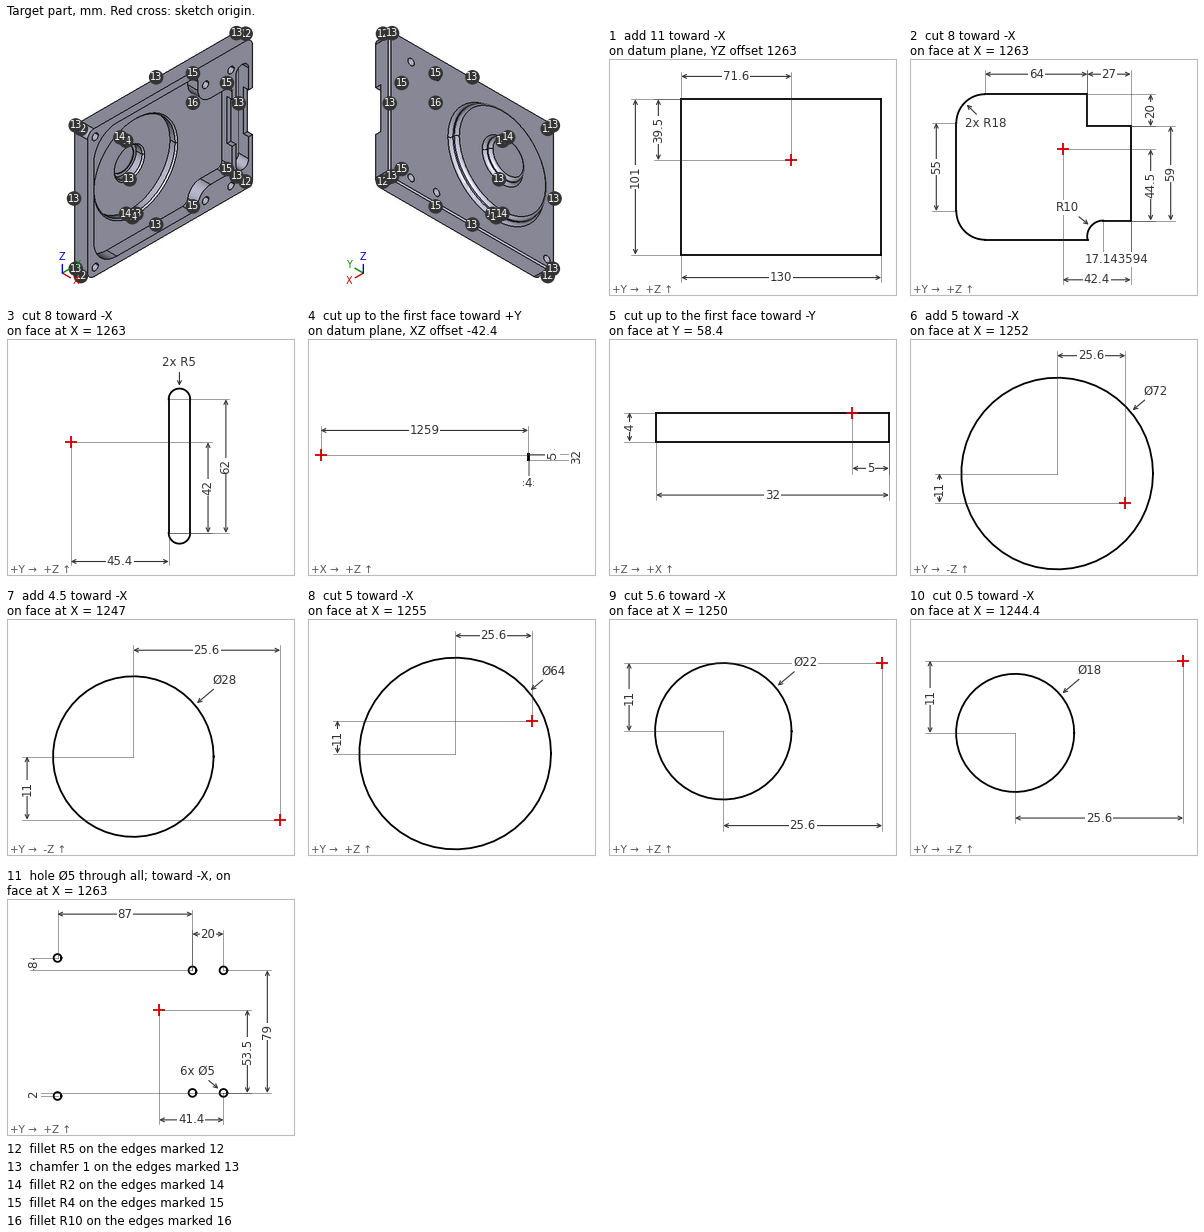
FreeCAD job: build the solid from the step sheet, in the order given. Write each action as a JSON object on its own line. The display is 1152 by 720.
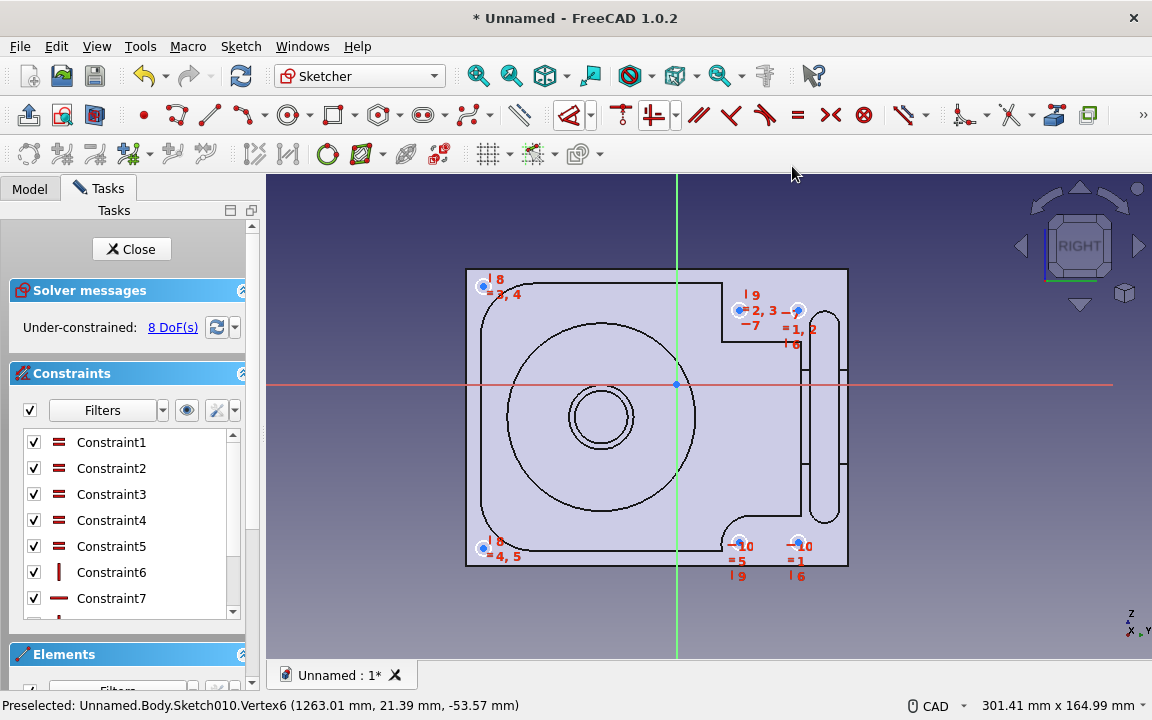
{"action": "scroll", "coordinate": [804, 548], "scroll_direction": "up", "scroll_amount": 5}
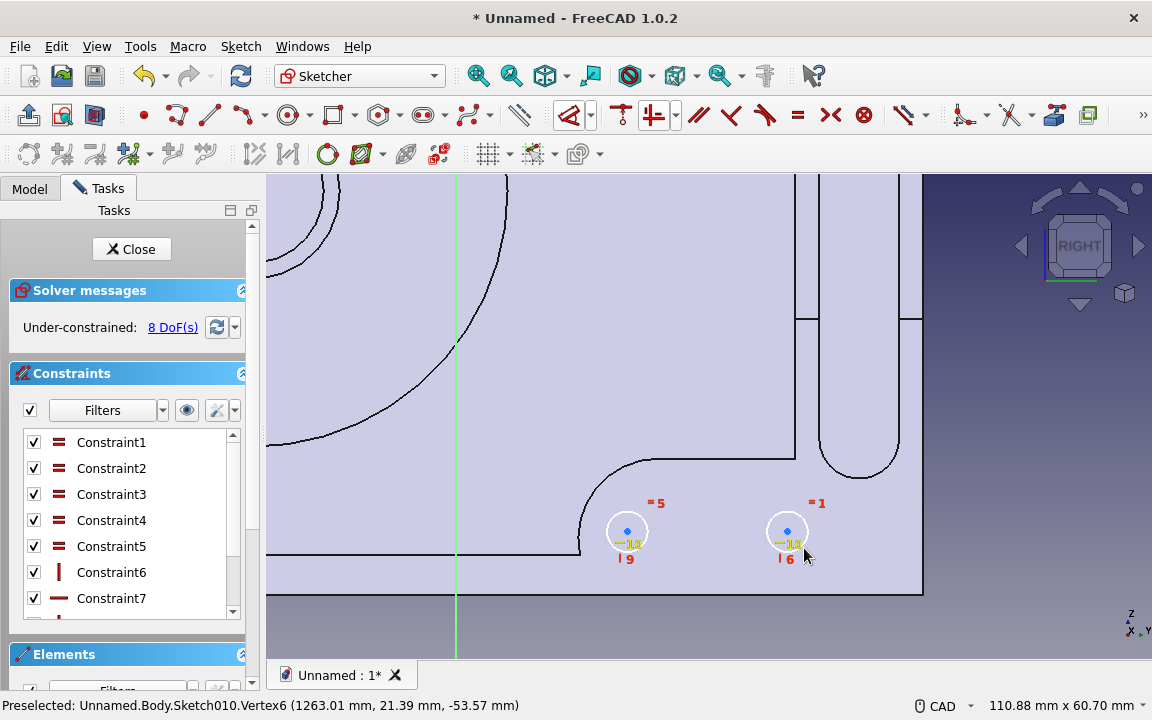
{"action": "left_click", "coordinate": [802, 546]}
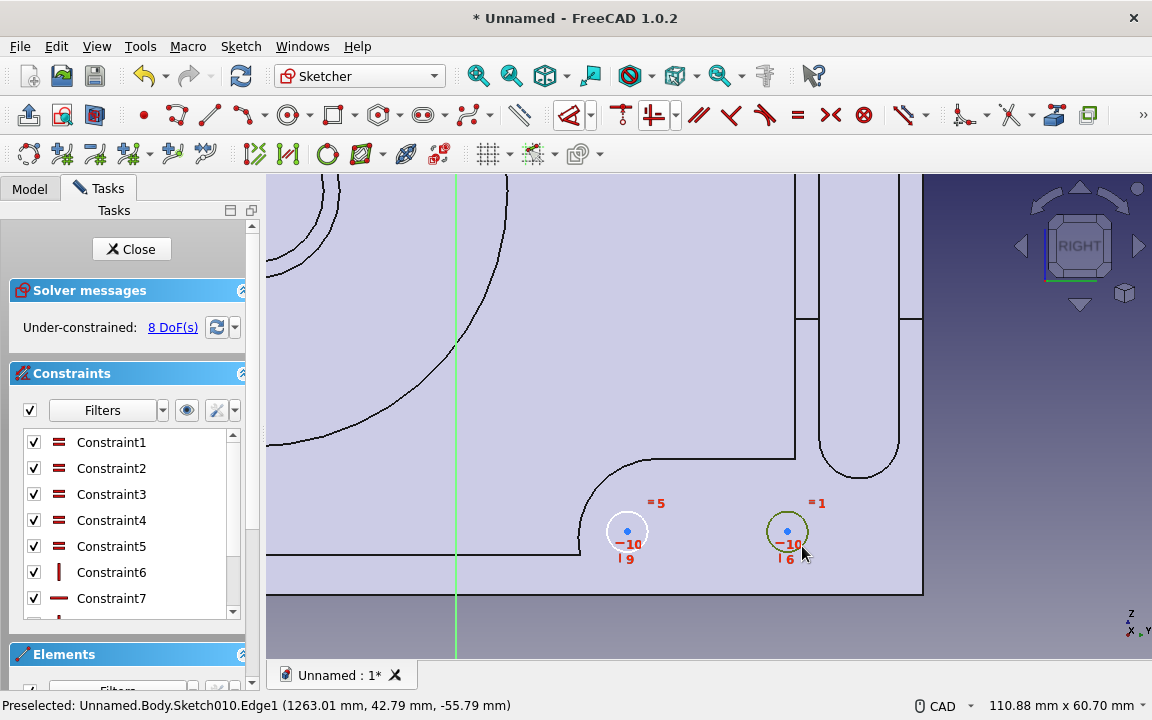
{"action": "key", "text": "k o"}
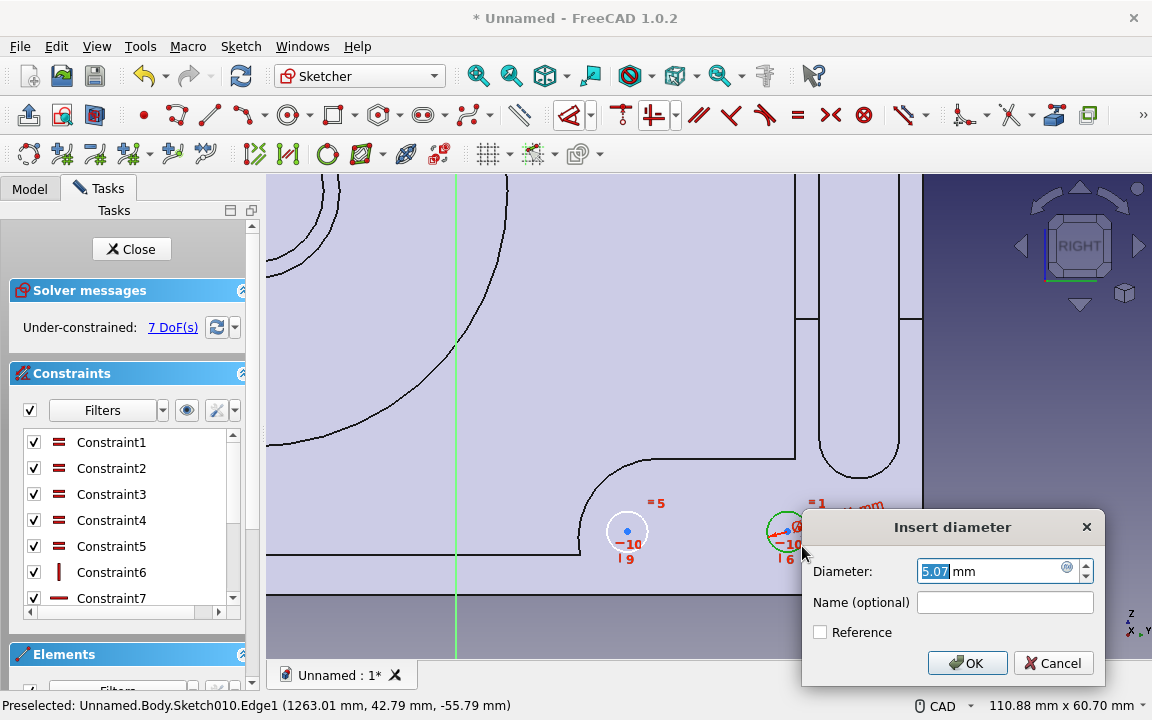
{"action": "type", "text": "5"}
{"action": "key", "text": "Return"}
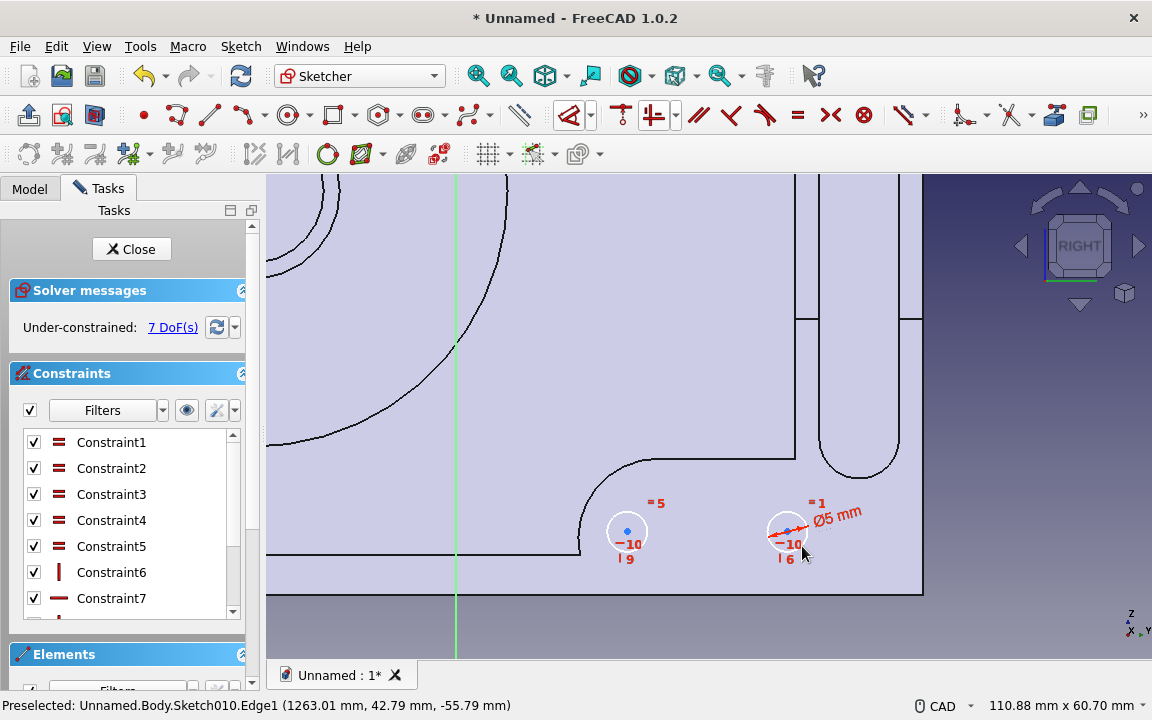
{"action": "scroll", "coordinate": [804, 548], "scroll_direction": "down", "scroll_amount": 5}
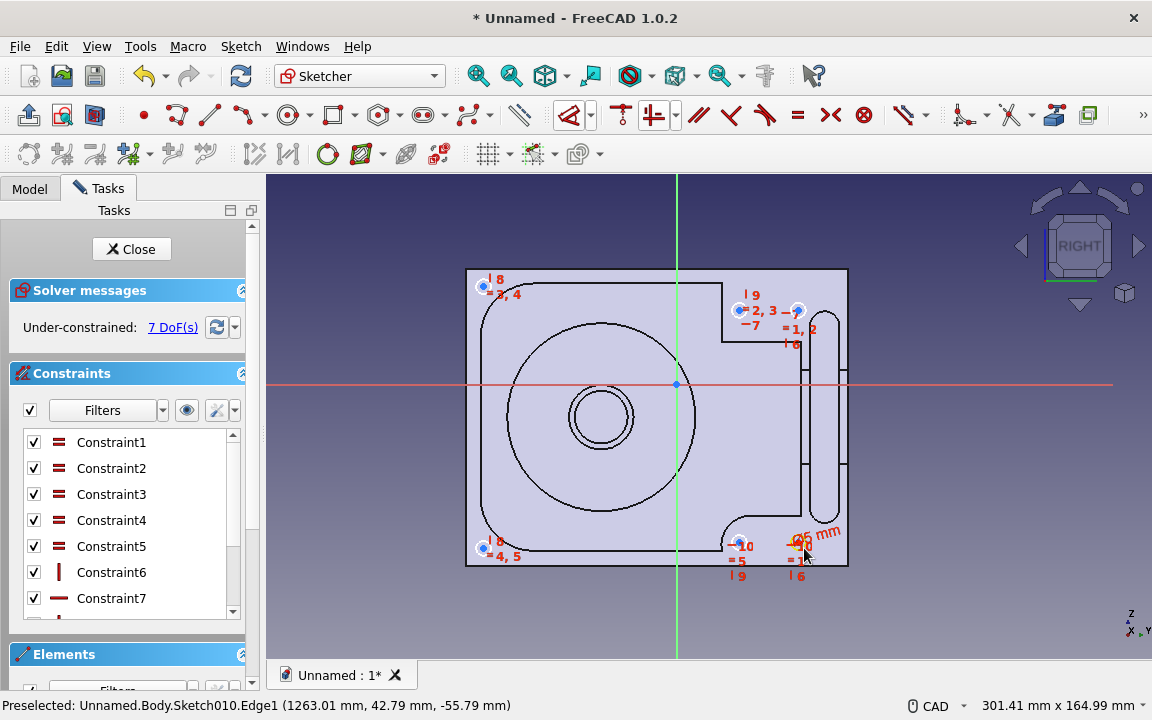
{"action": "scroll", "coordinate": [739, 310], "scroll_direction": "up", "scroll_amount": 3}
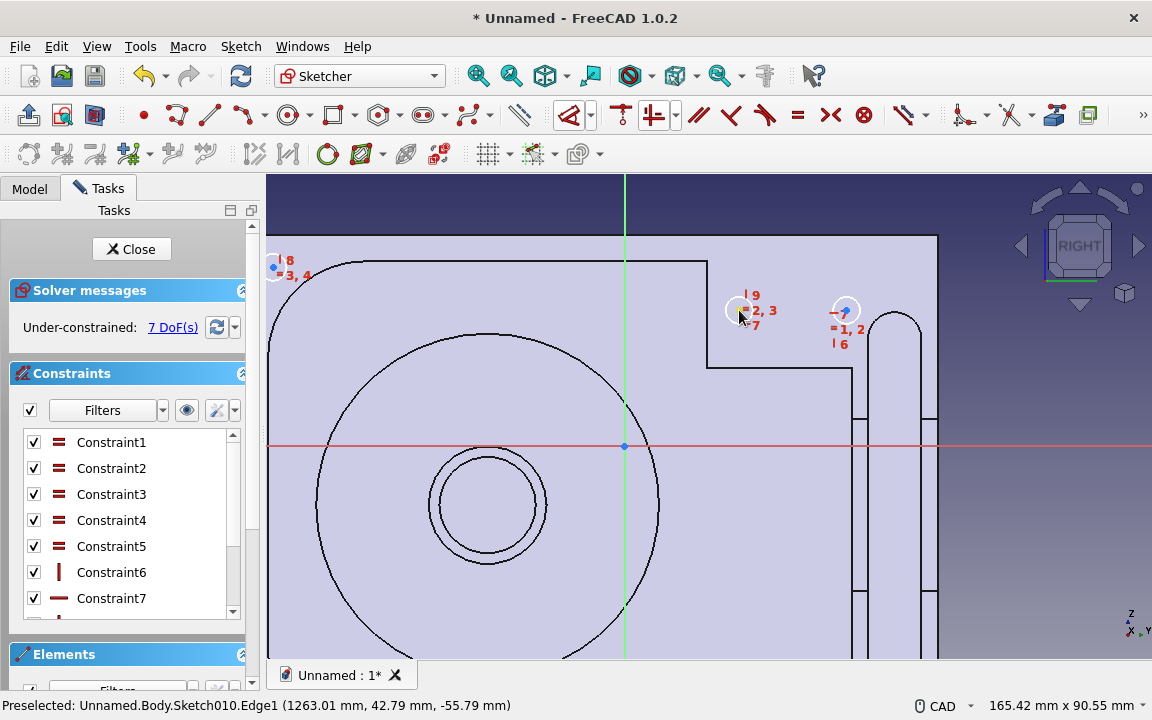
{"action": "left_click", "coordinate": [739, 310]}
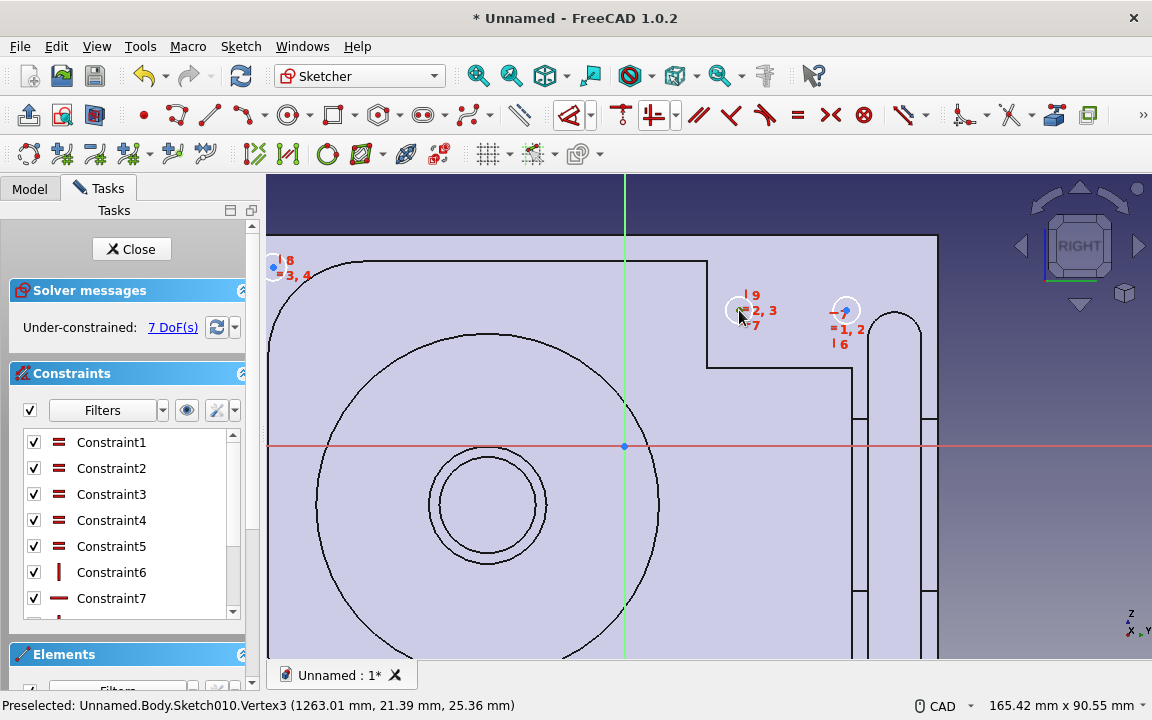
{"action": "scroll", "coordinate": [739, 309], "scroll_direction": "down", "scroll_amount": 3}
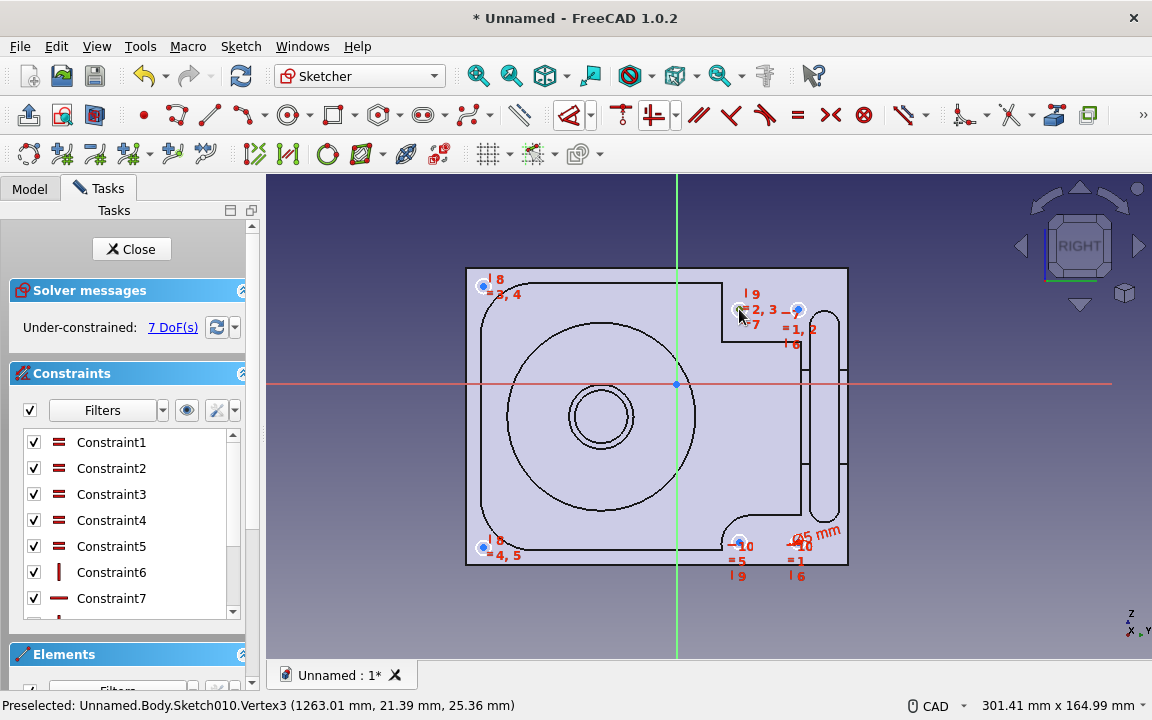
{"action": "scroll", "coordinate": [484, 286], "scroll_direction": "up", "scroll_amount": 3}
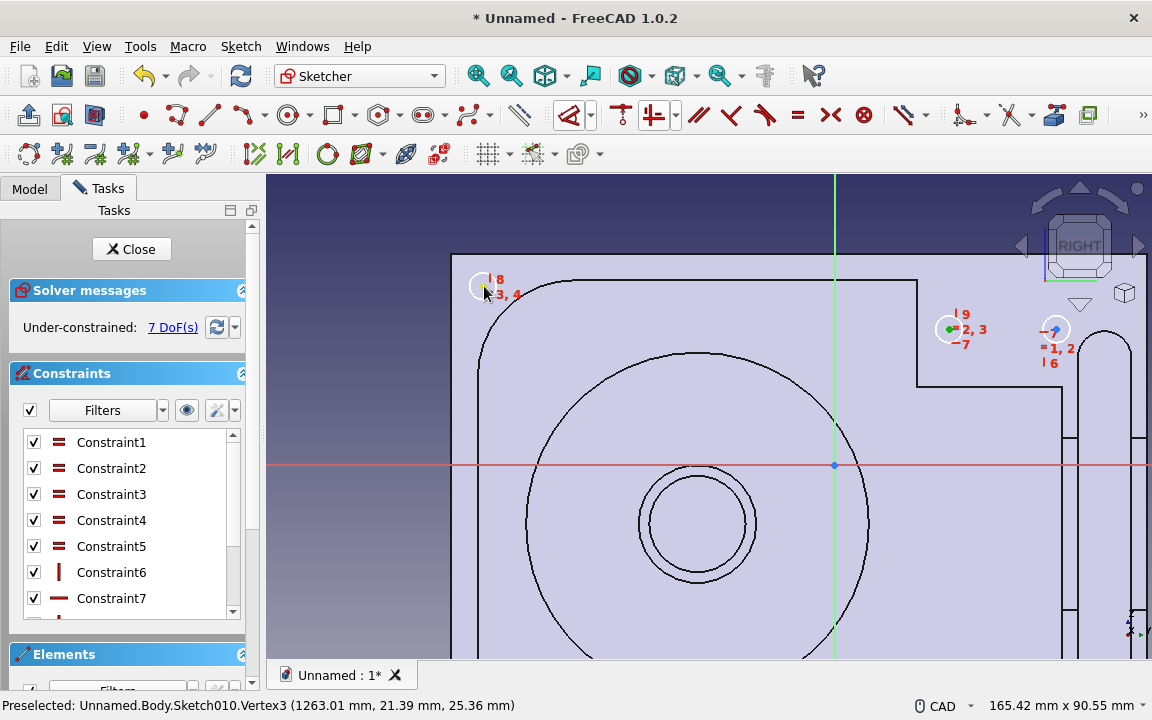
{"action": "left_click", "coordinate": [483, 286]}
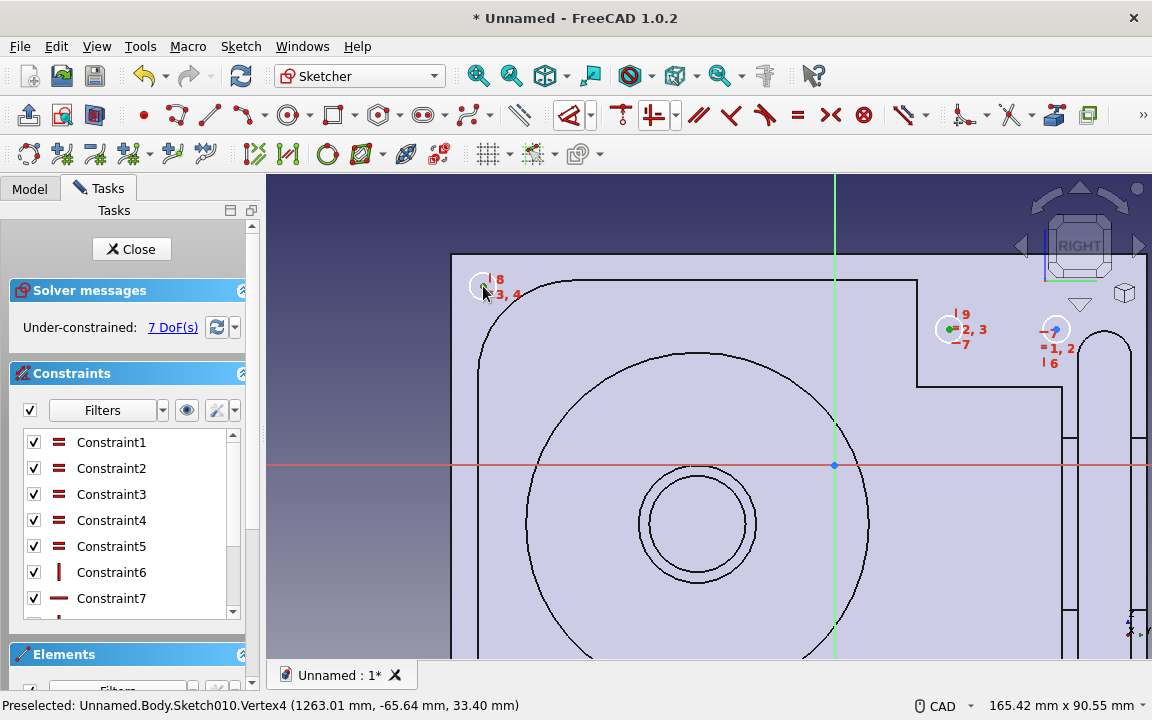
{"action": "left_click", "coordinate": [590, 116]}